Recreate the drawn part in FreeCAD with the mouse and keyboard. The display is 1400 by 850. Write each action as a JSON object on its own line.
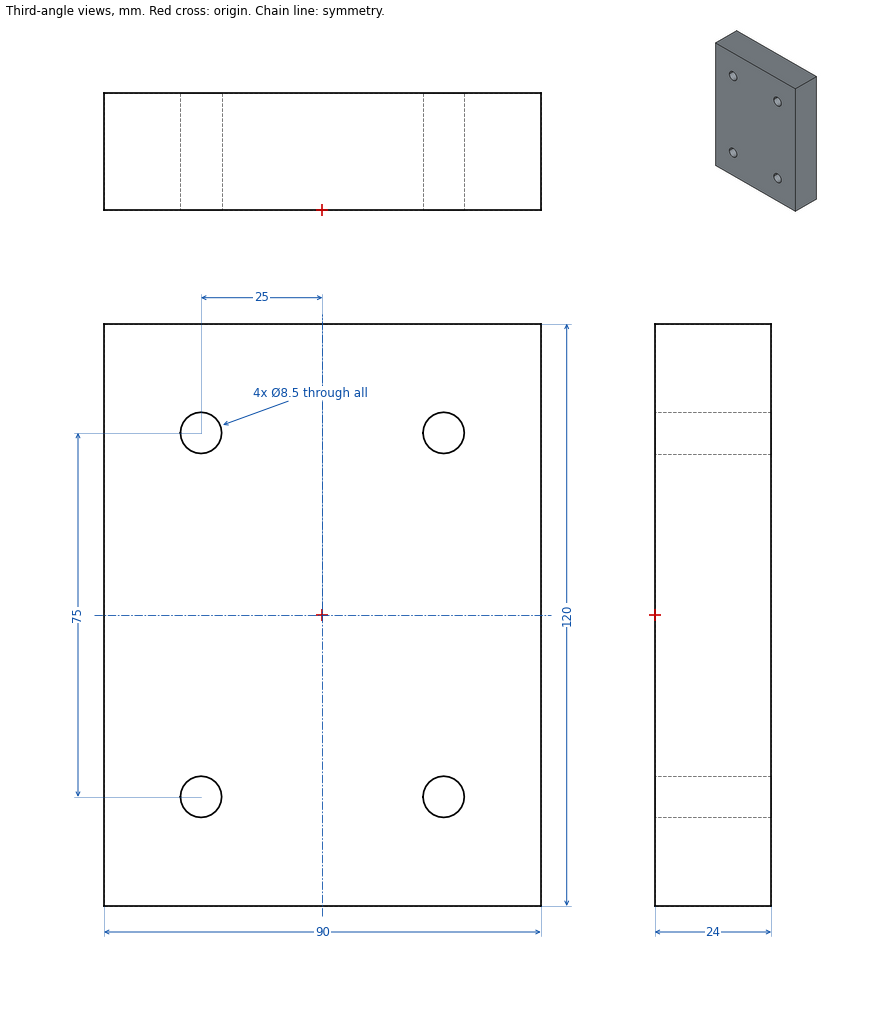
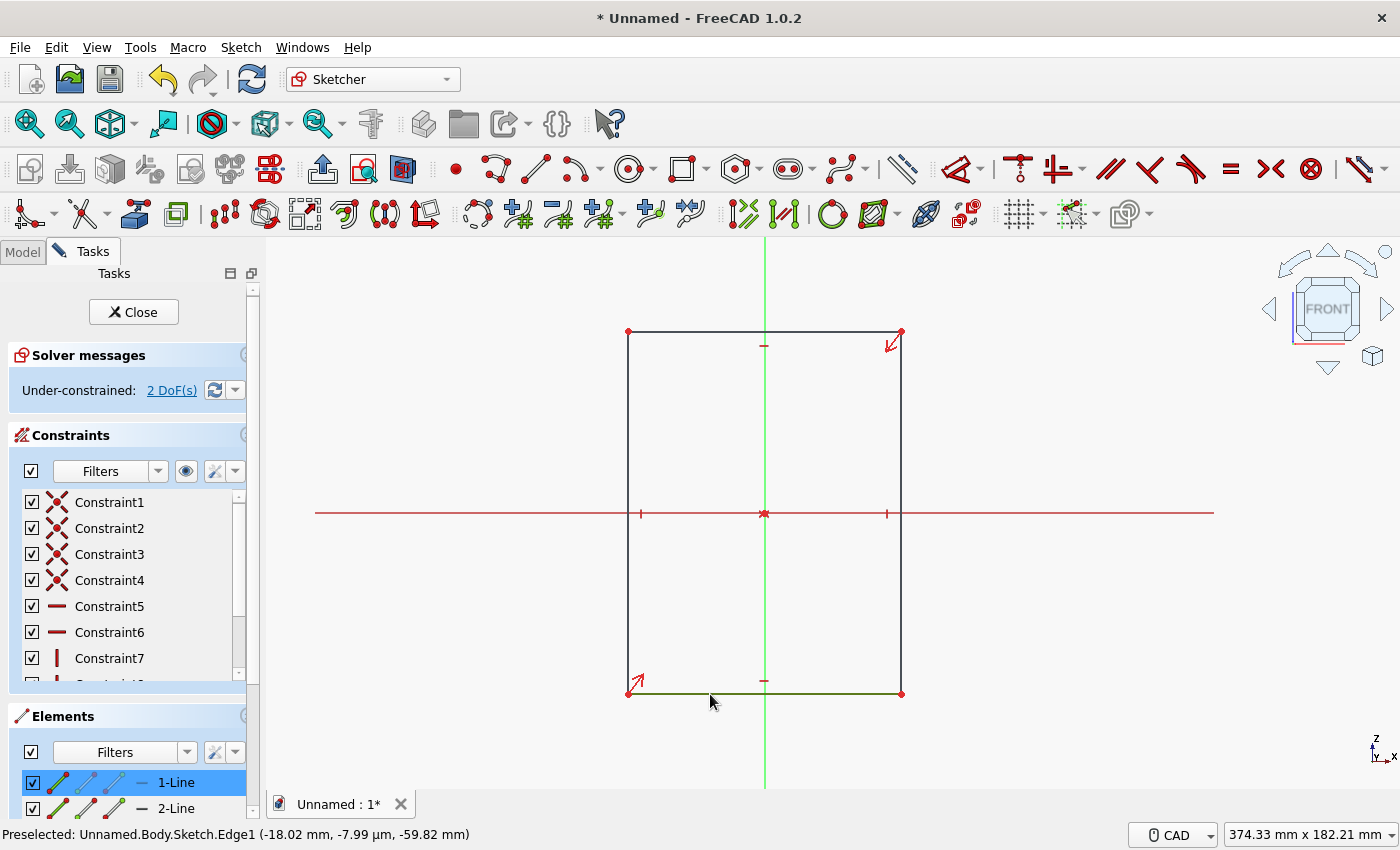
{"action": "key", "text": "l"}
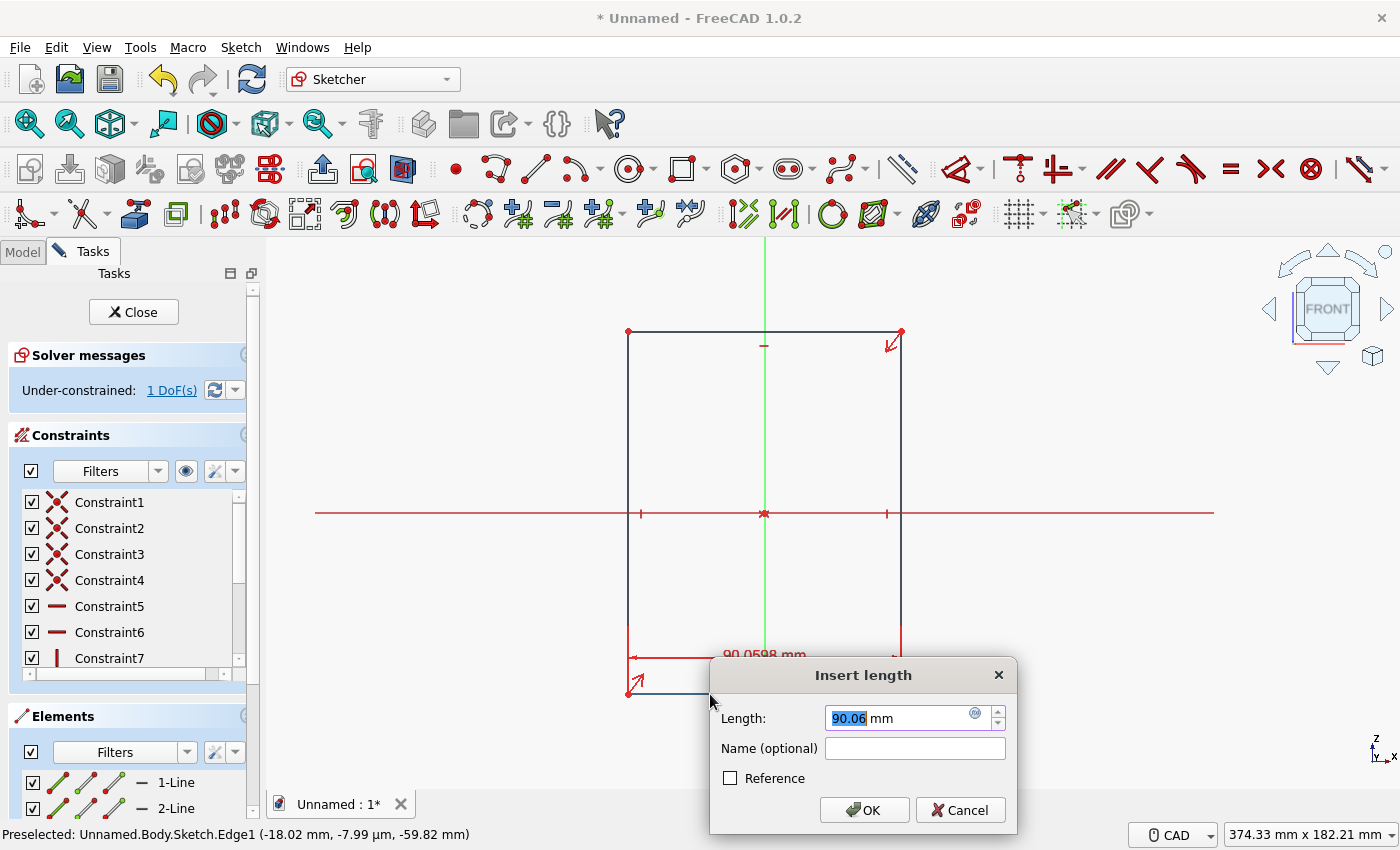
{"action": "type", "text": "90"}
{"action": "key", "text": "Return"}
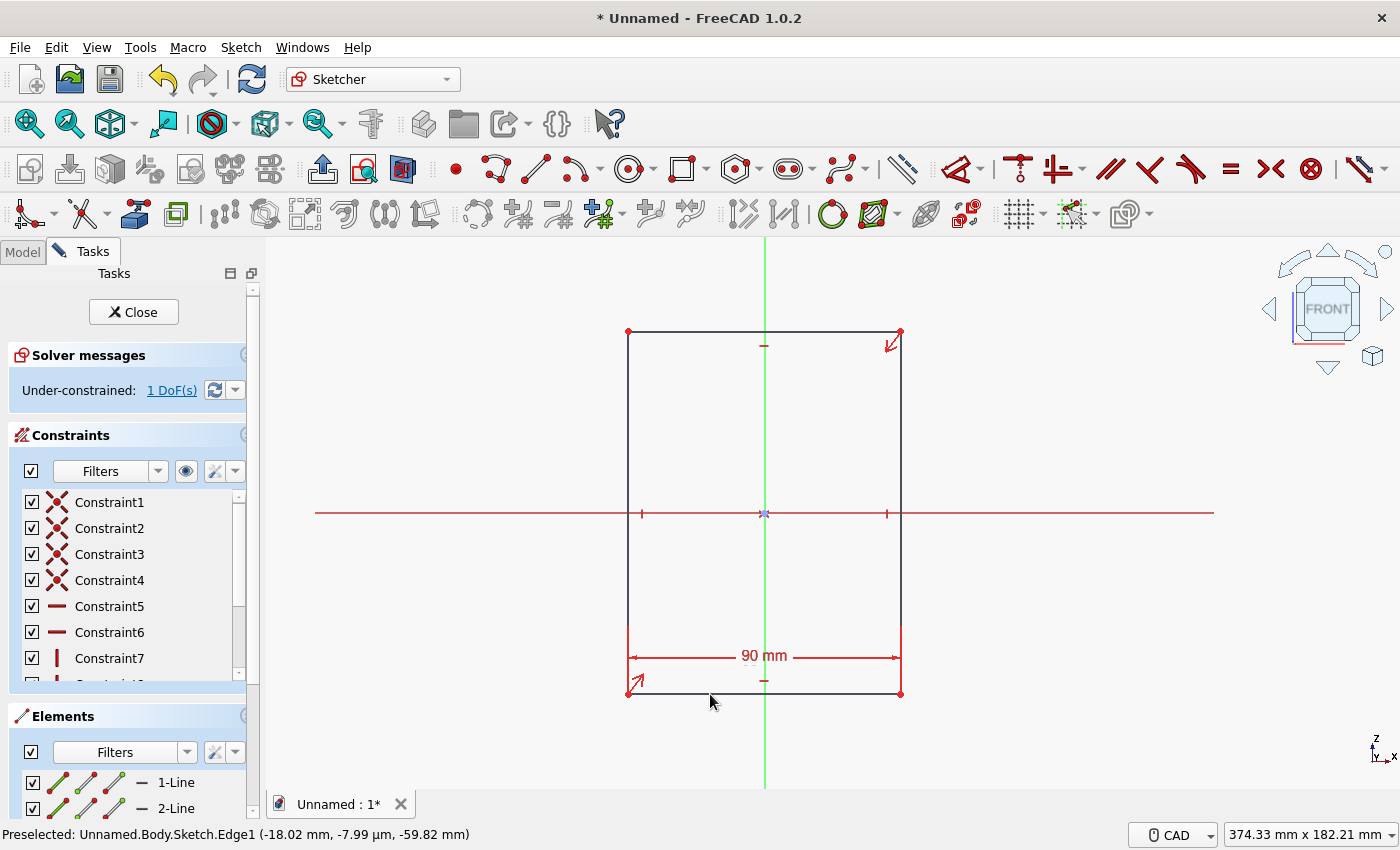
{"action": "left_click", "coordinate": [901, 586]}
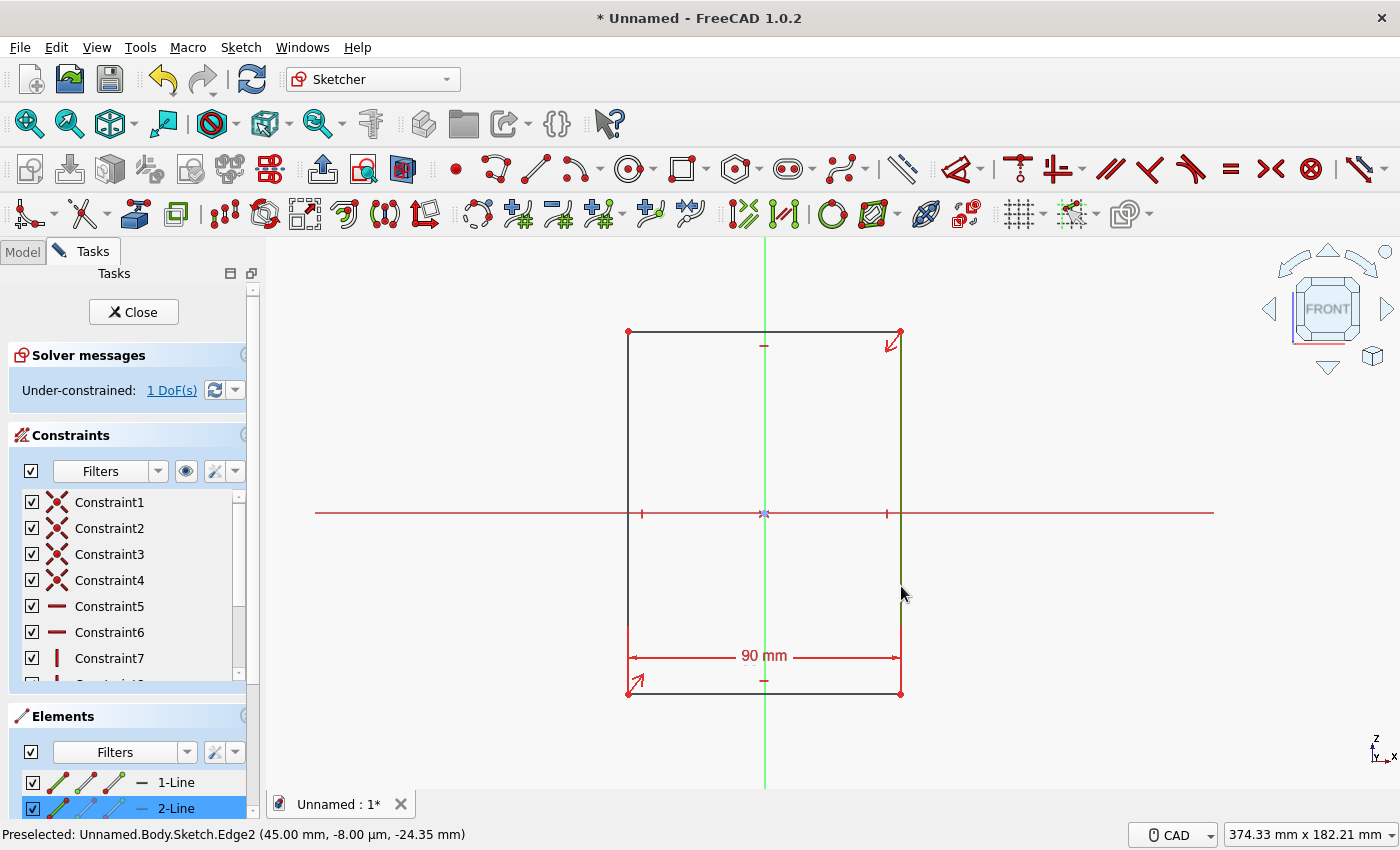
{"action": "key", "text": "i"}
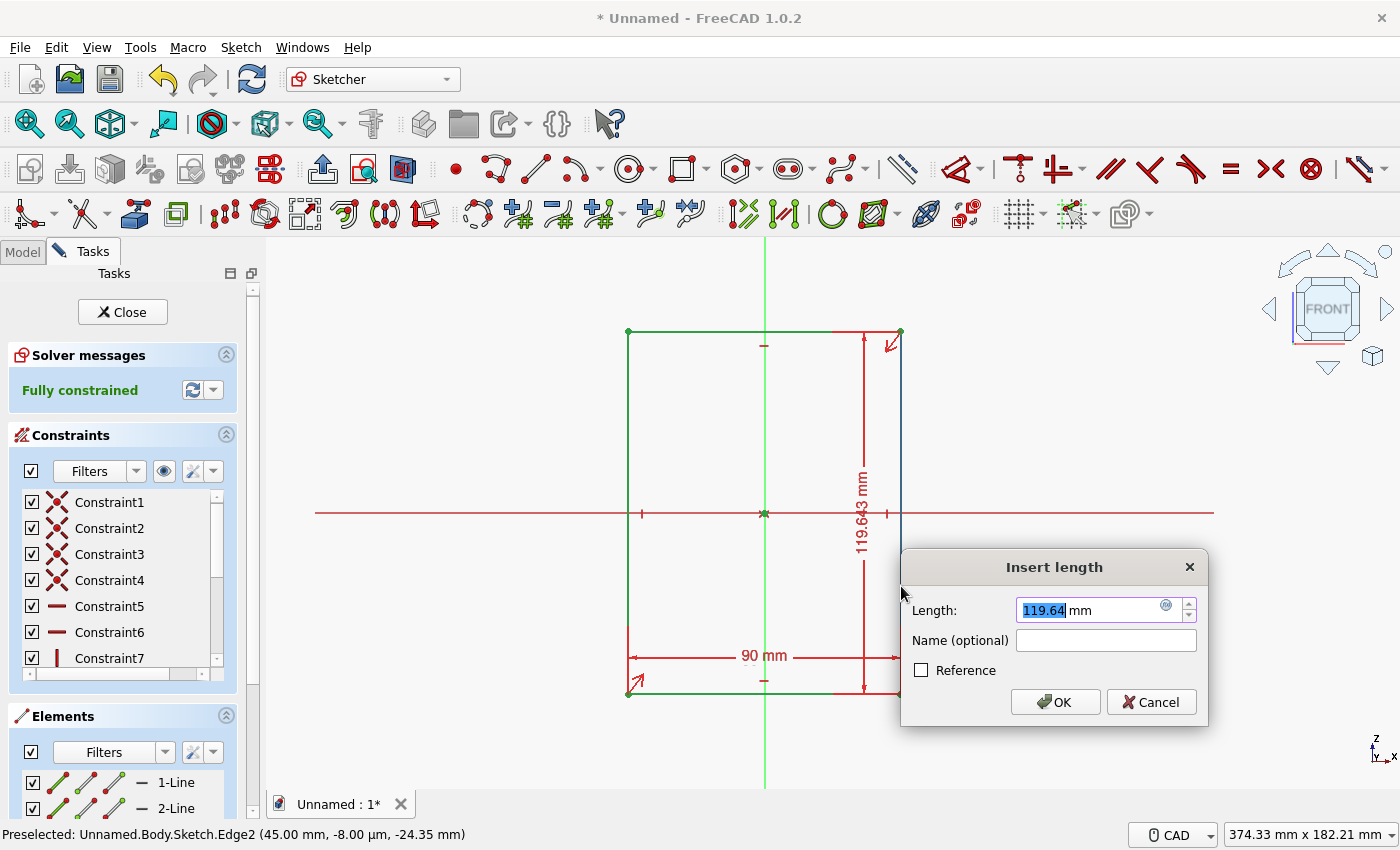
{"action": "type", "text": "120"}
{"action": "key", "text": "Return"}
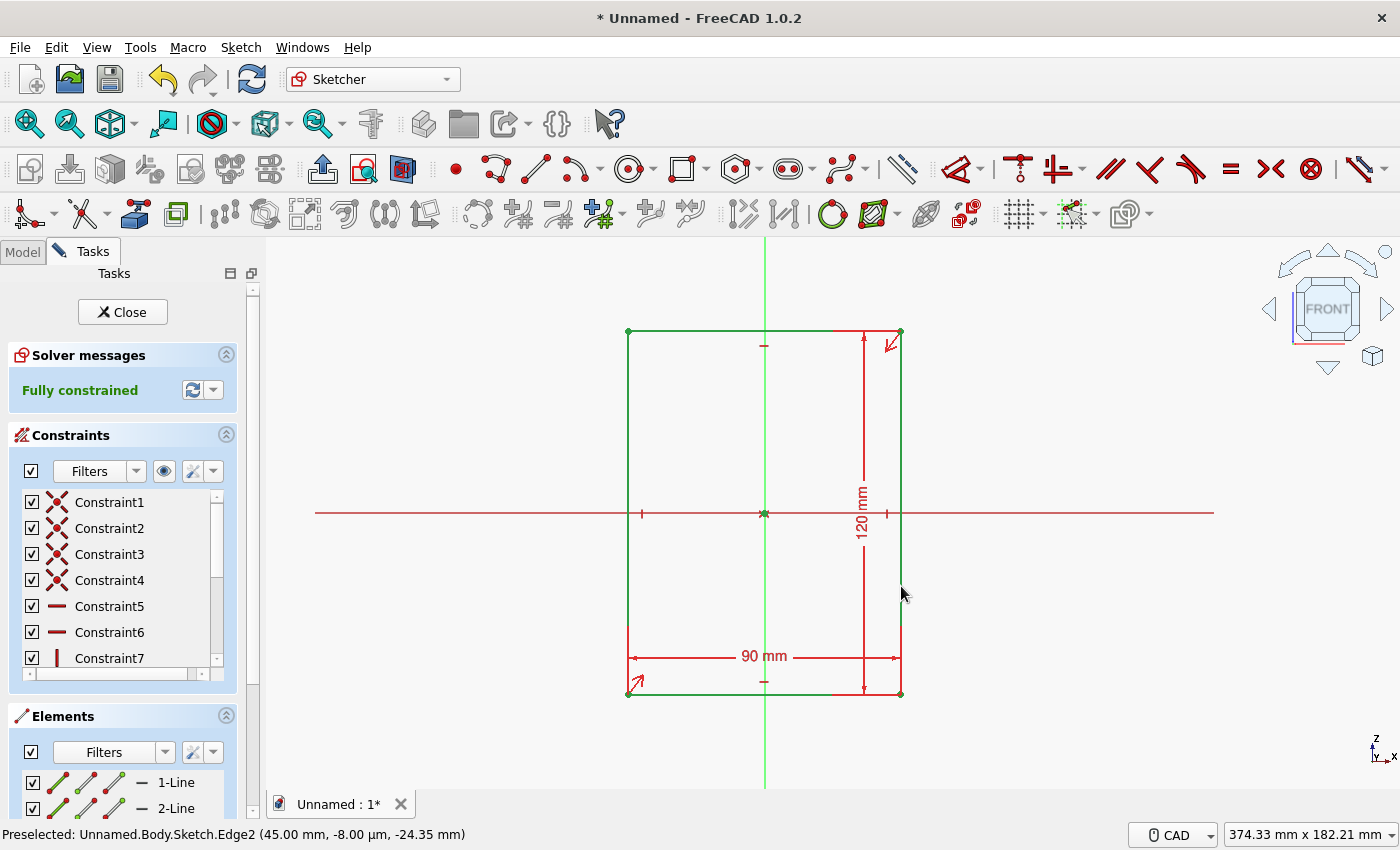
{"action": "left_click", "coordinate": [123, 312]}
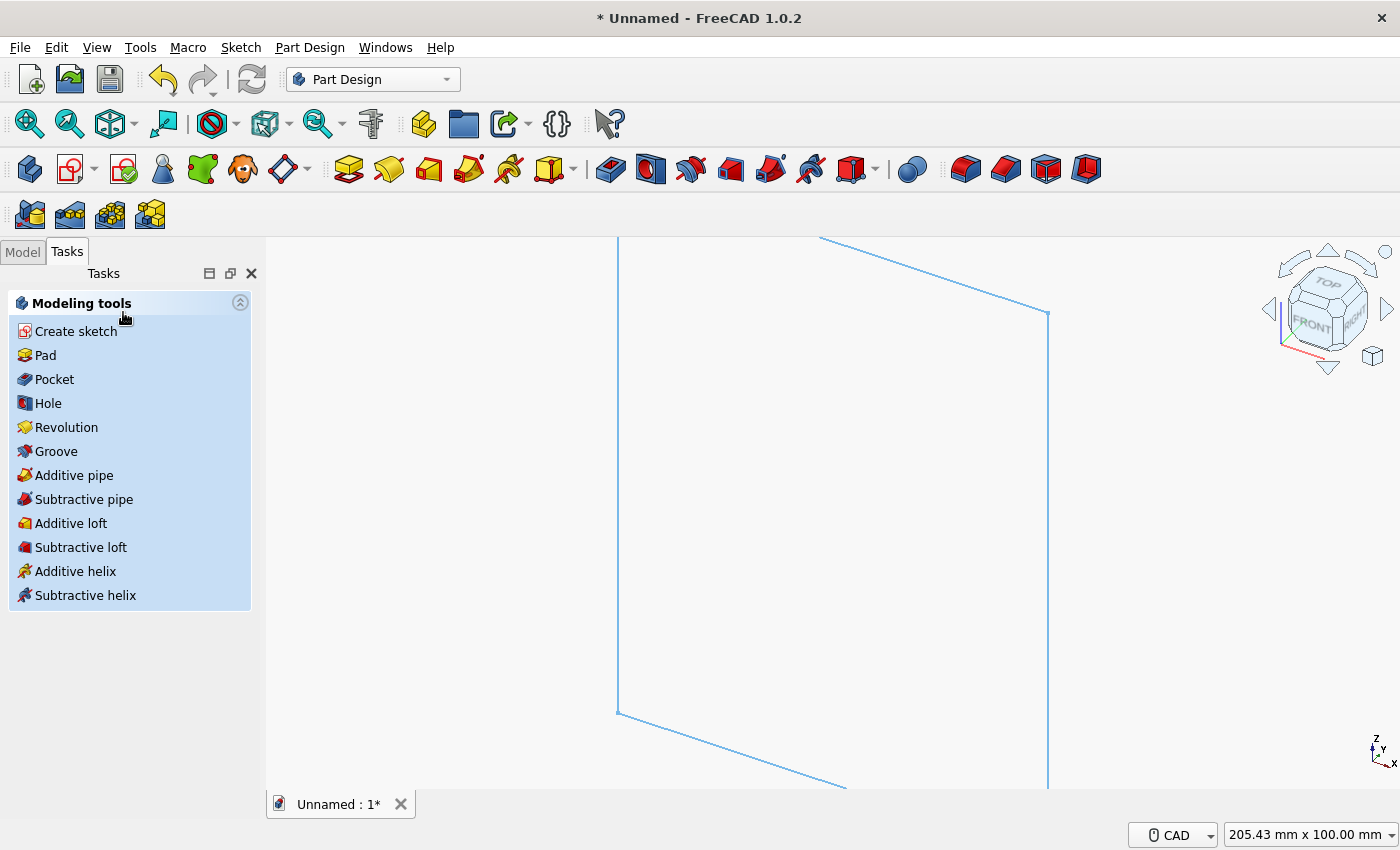
{"action": "left_click", "coordinate": [350, 170]}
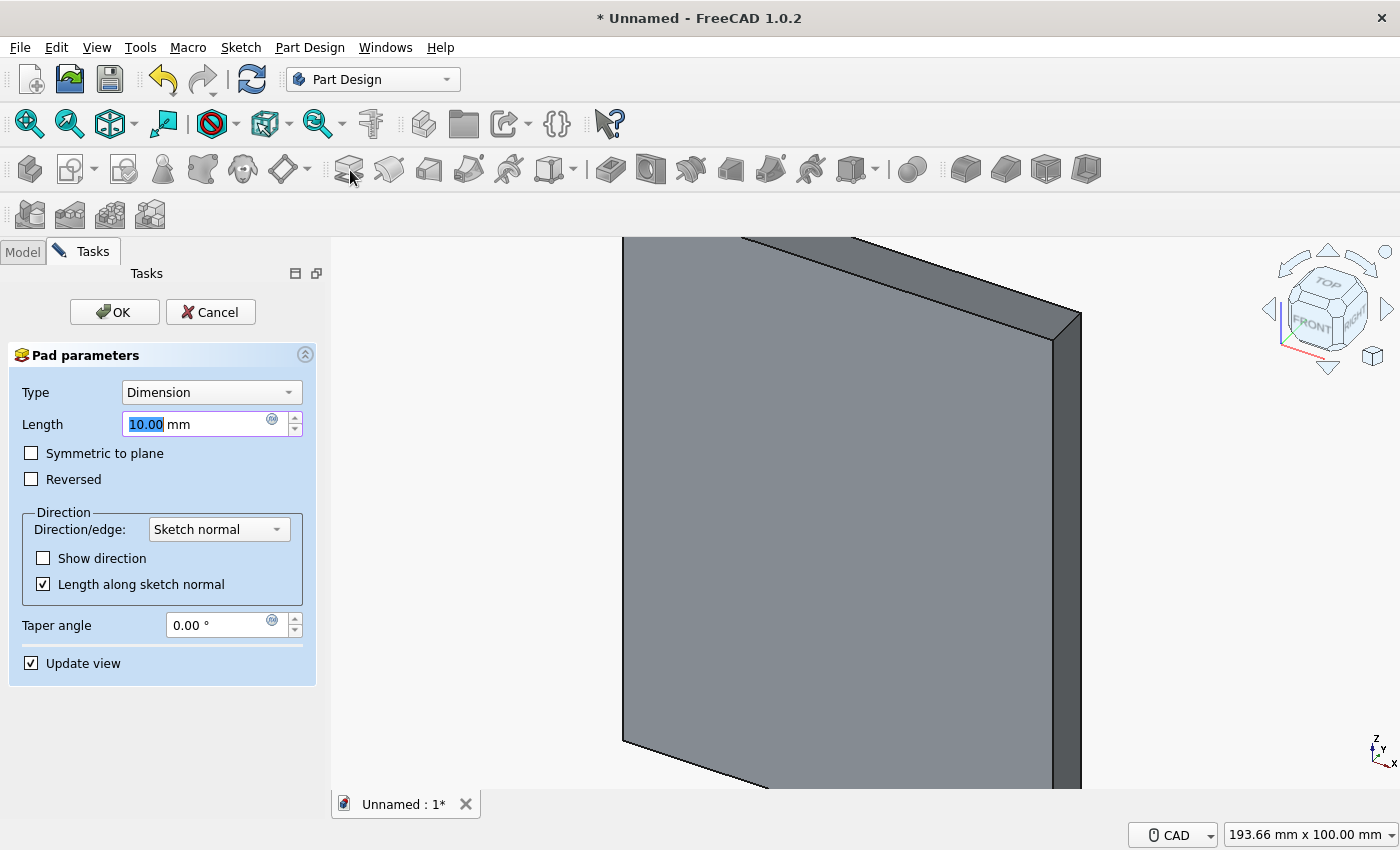
{"action": "type", "text": "24"}
{"action": "key", "text": "Tab"}